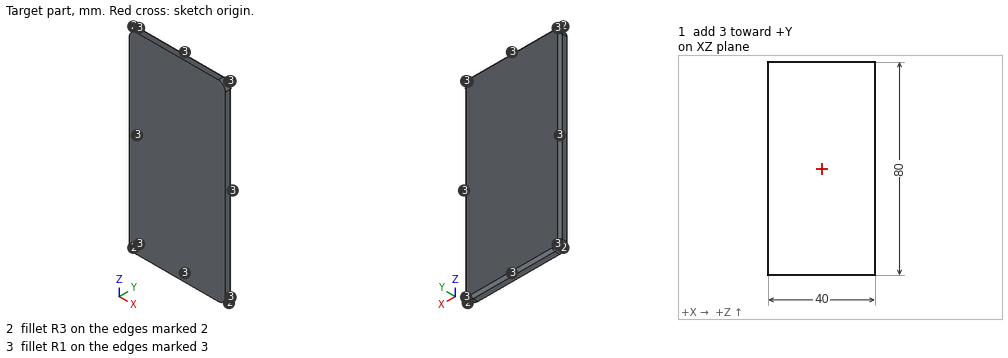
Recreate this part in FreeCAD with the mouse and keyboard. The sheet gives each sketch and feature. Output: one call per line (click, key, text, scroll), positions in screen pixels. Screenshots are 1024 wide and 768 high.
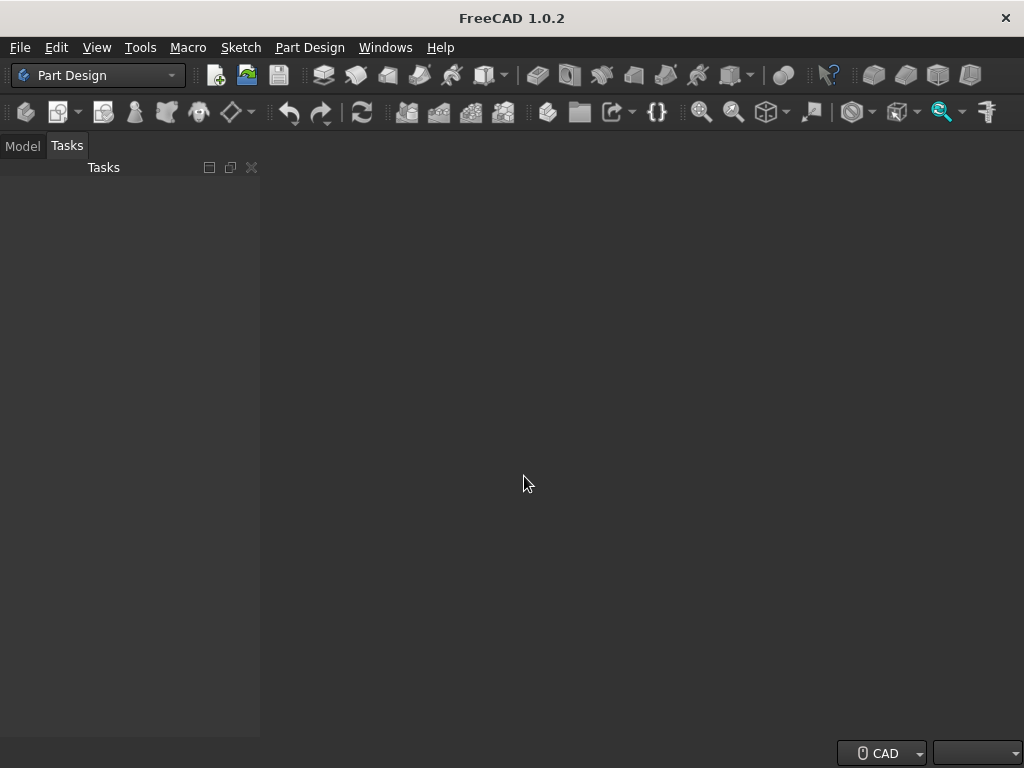
key(ctrl+n)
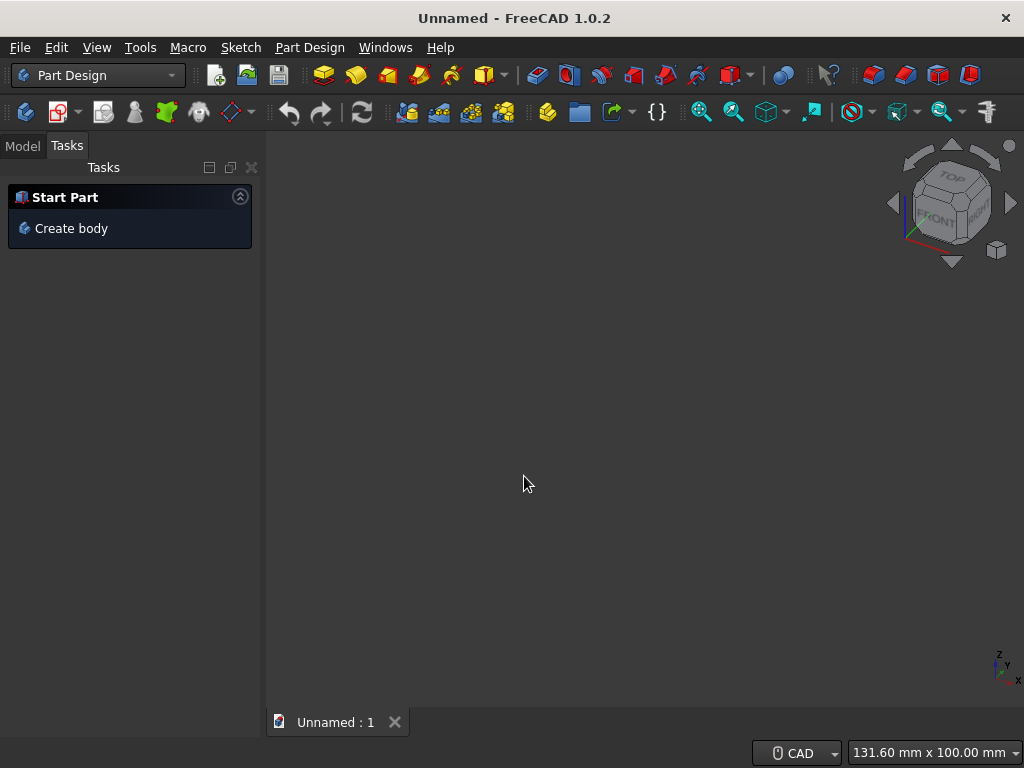
click(58, 112)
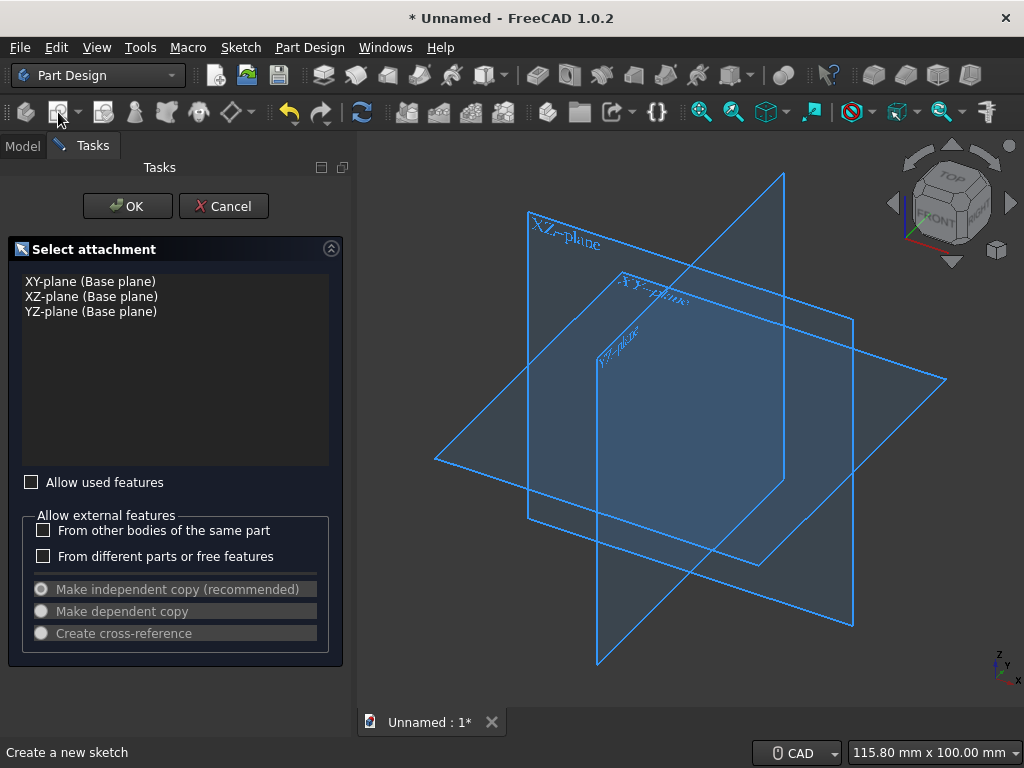
click(82, 296)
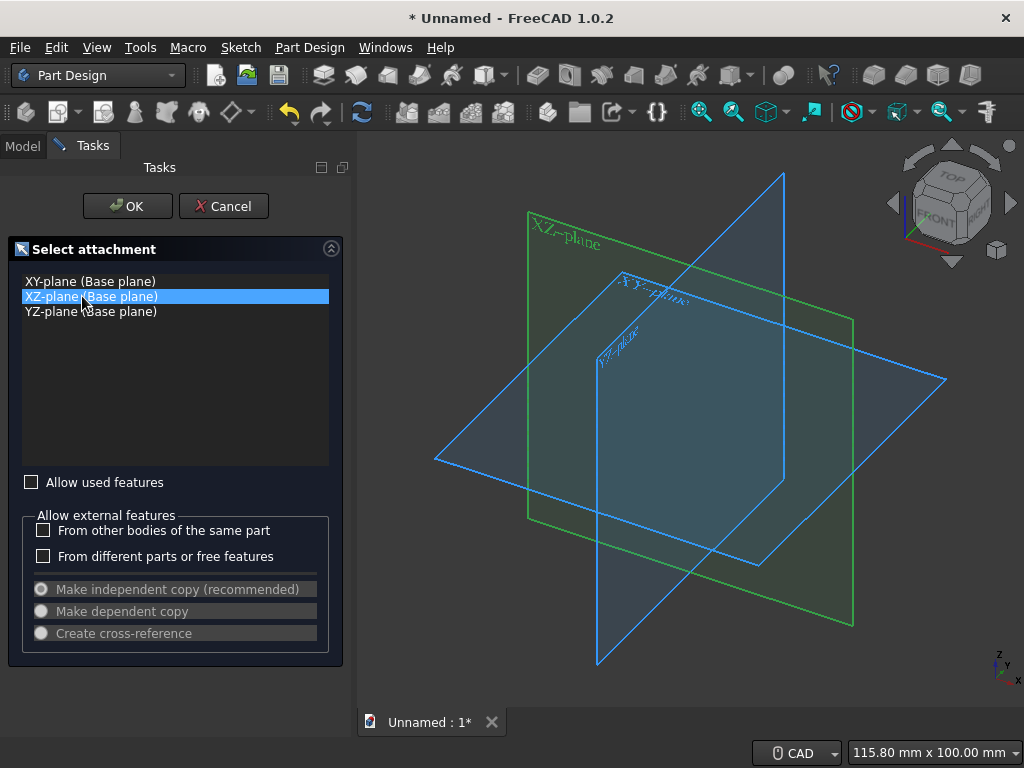
click(128, 206)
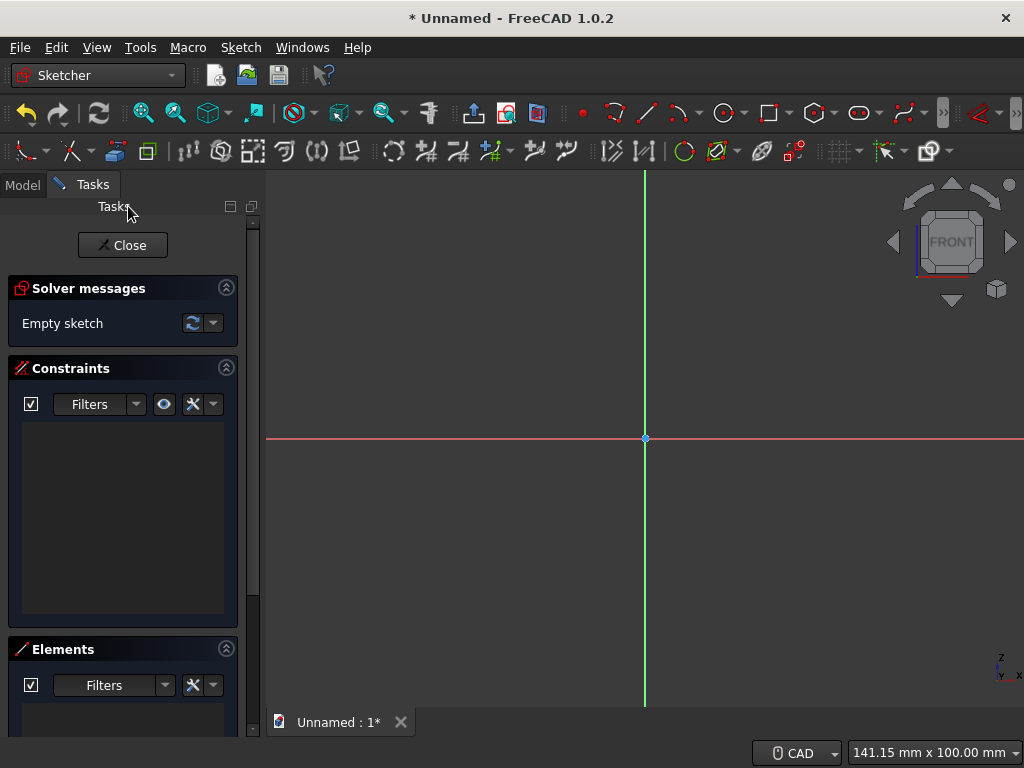
click(792, 114)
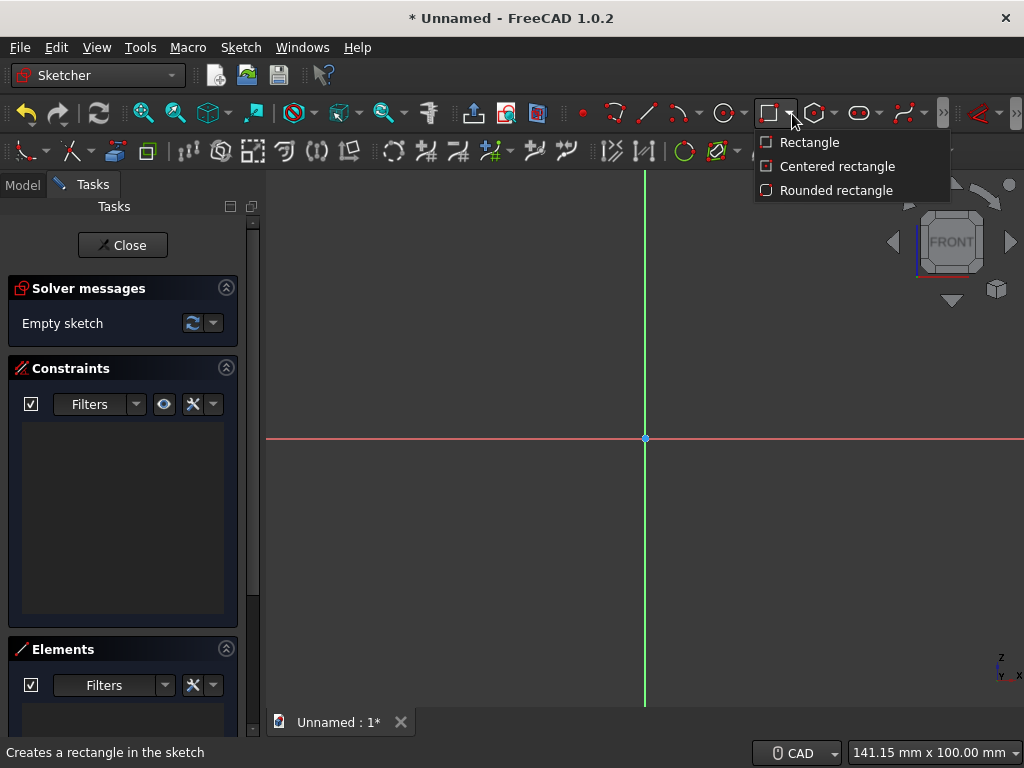
click(852, 166)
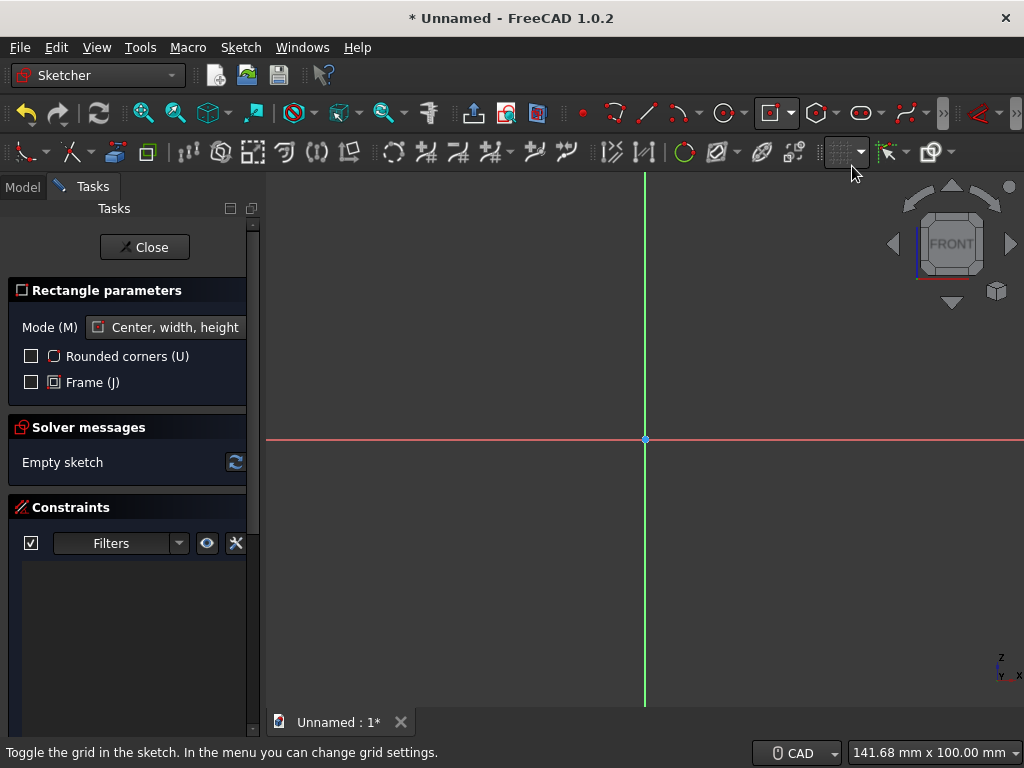
click(645, 440)
move(752, 226)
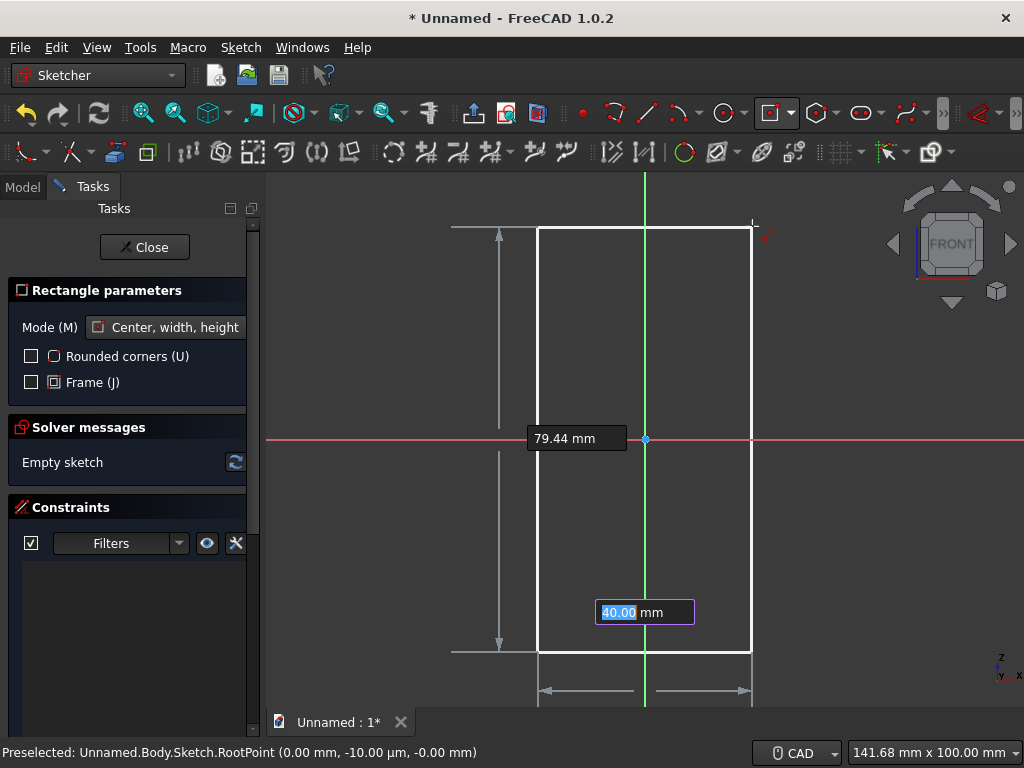
text(40)
key(Tab)
text(80)
key(Return)
key(Escape)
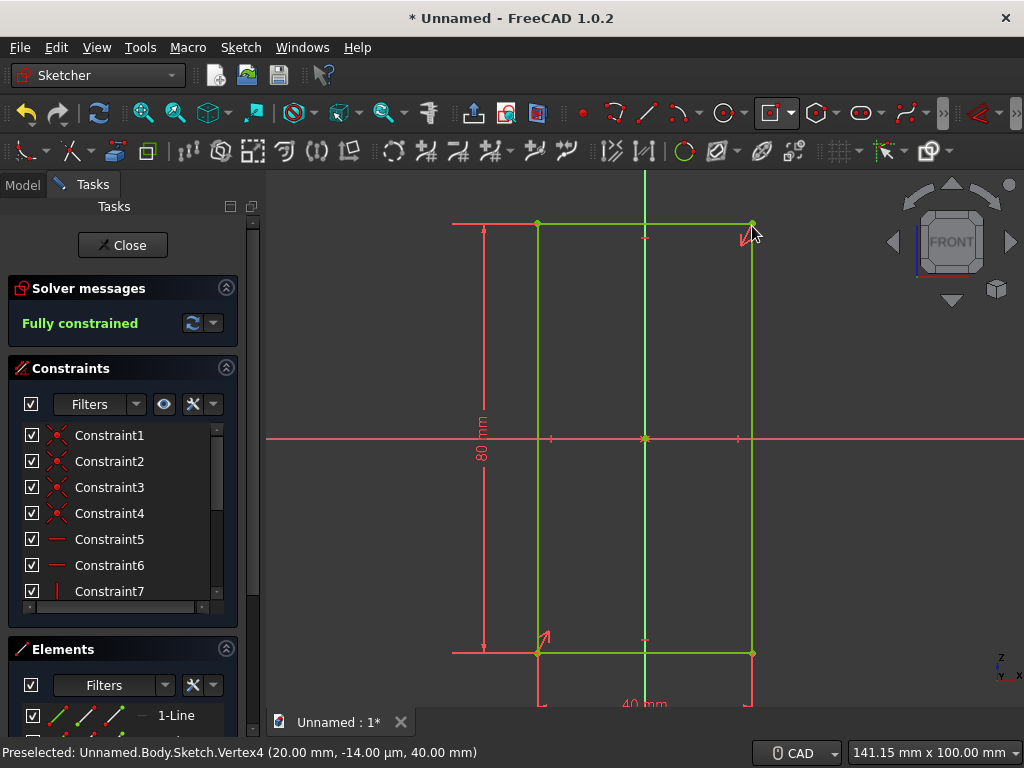
click(123, 245)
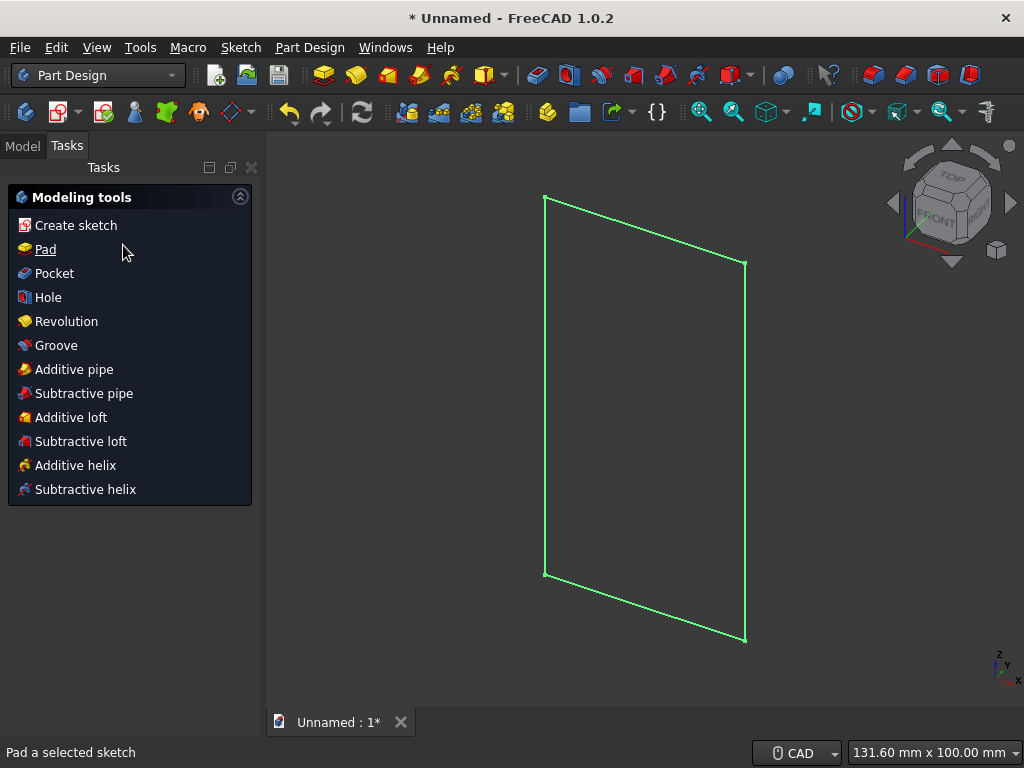
click(324, 76)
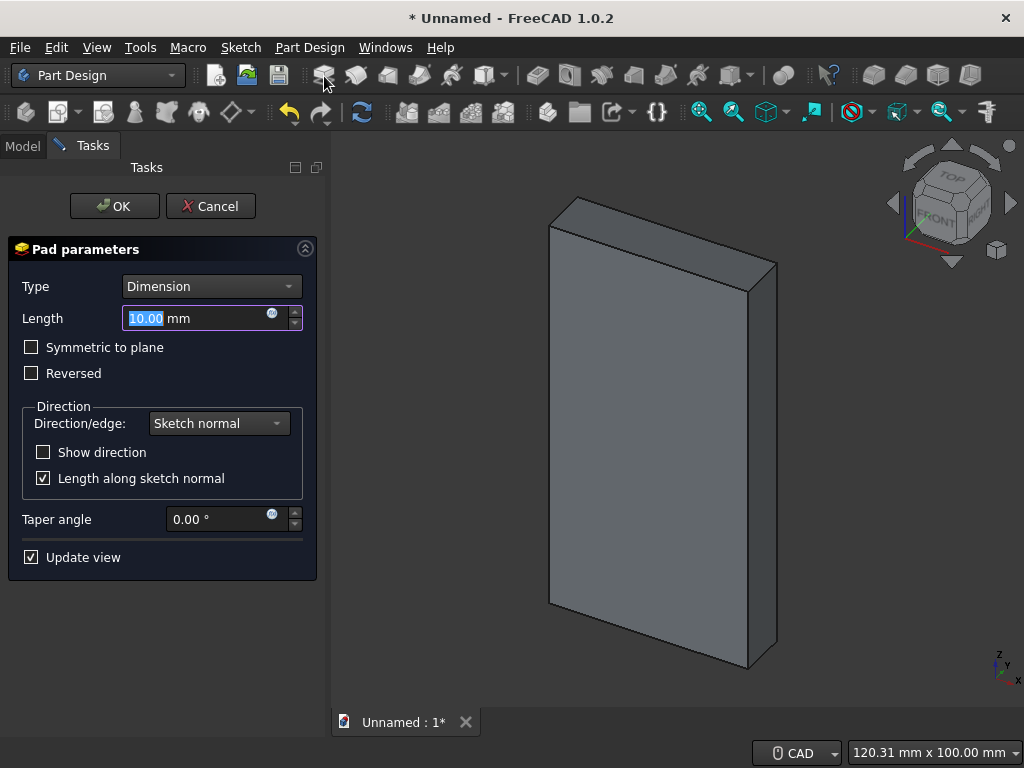
text(3)
key(Tab)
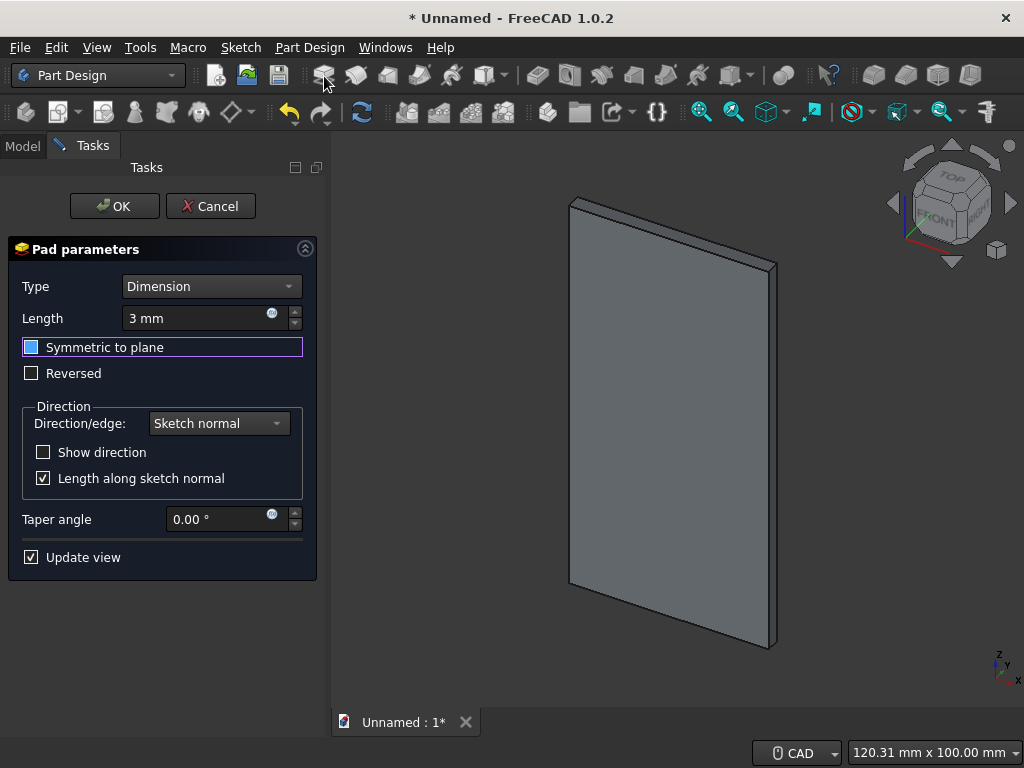
click(30, 373)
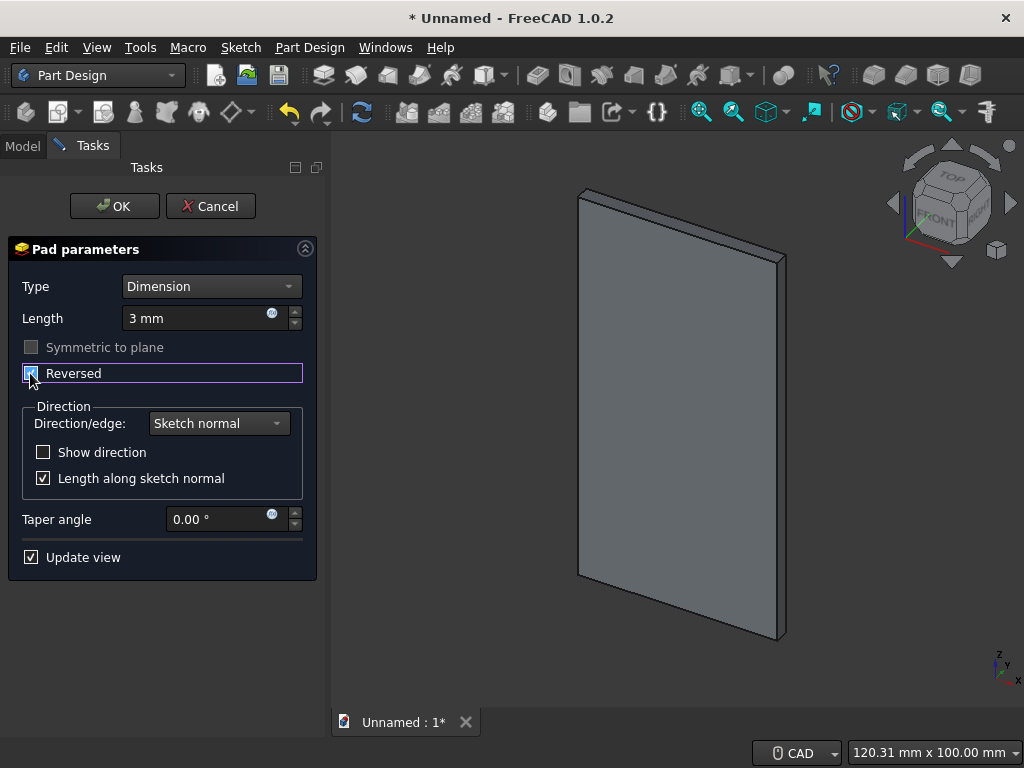
click(115, 206)